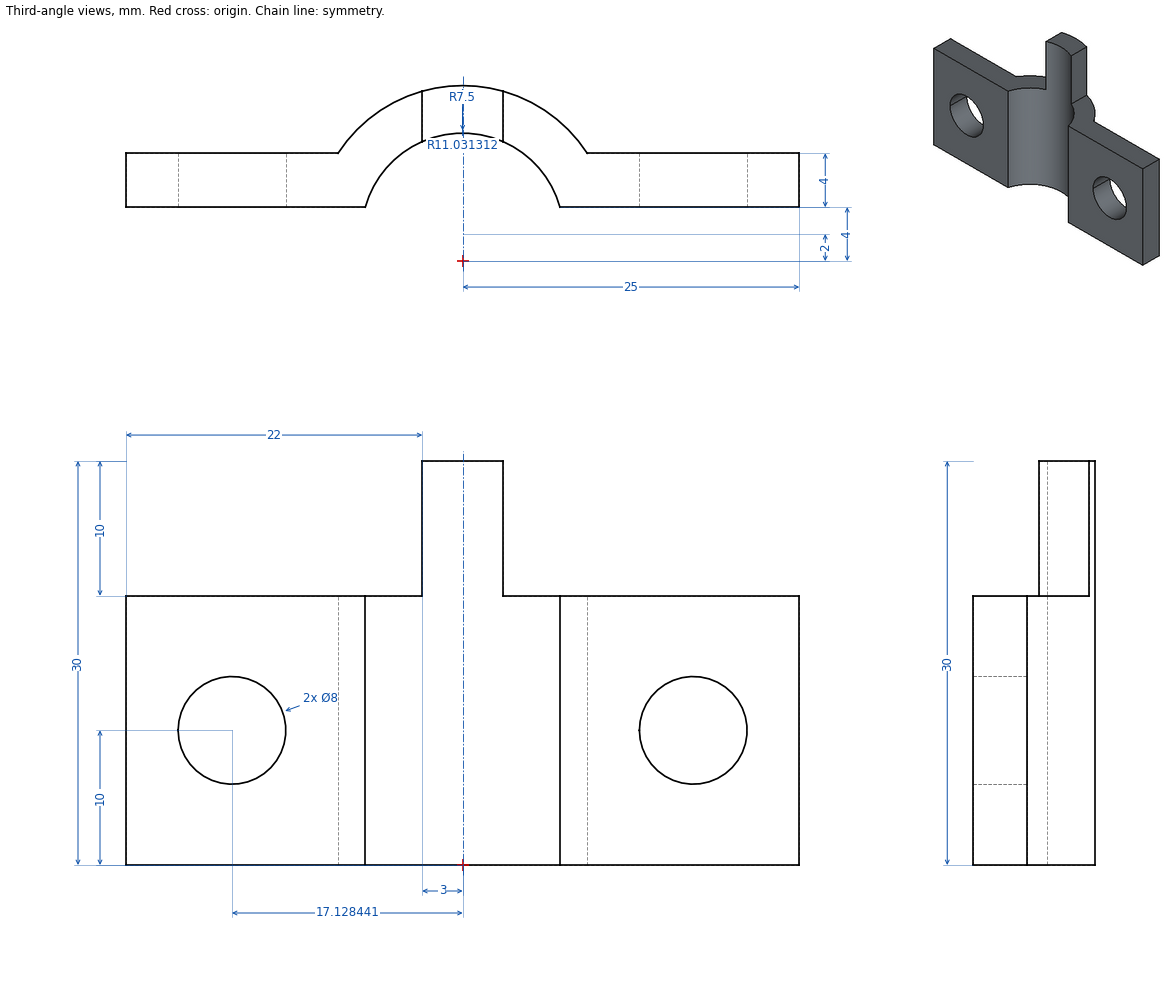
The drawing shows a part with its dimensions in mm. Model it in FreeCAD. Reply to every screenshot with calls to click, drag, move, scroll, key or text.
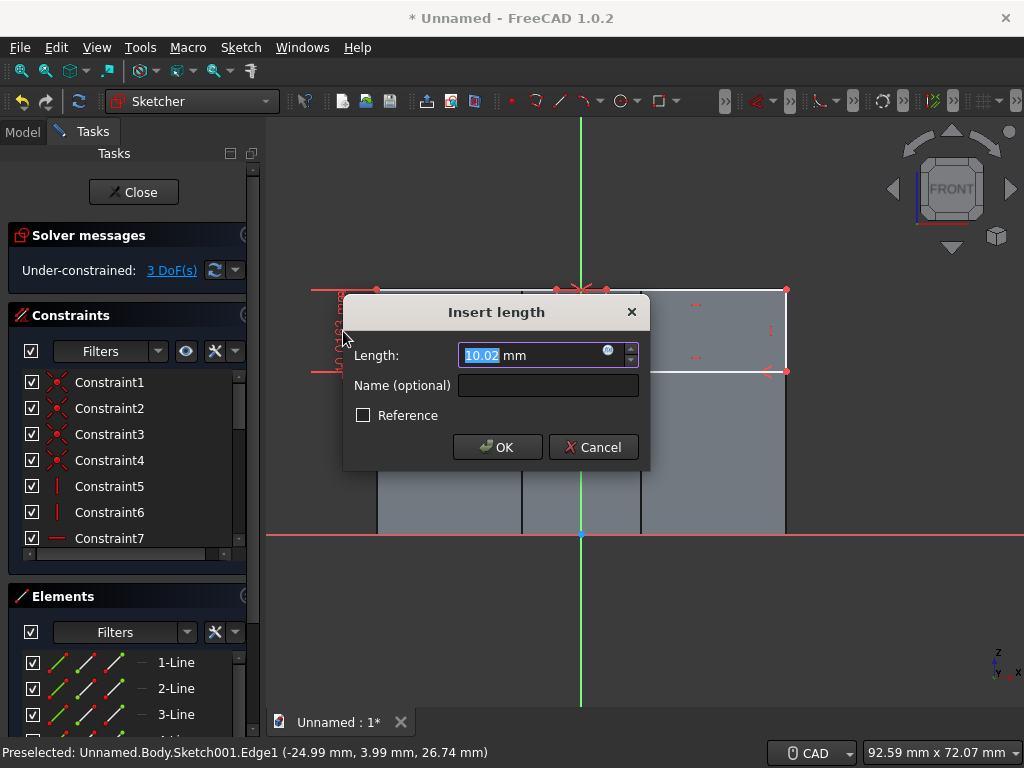
text(10)
key(Return)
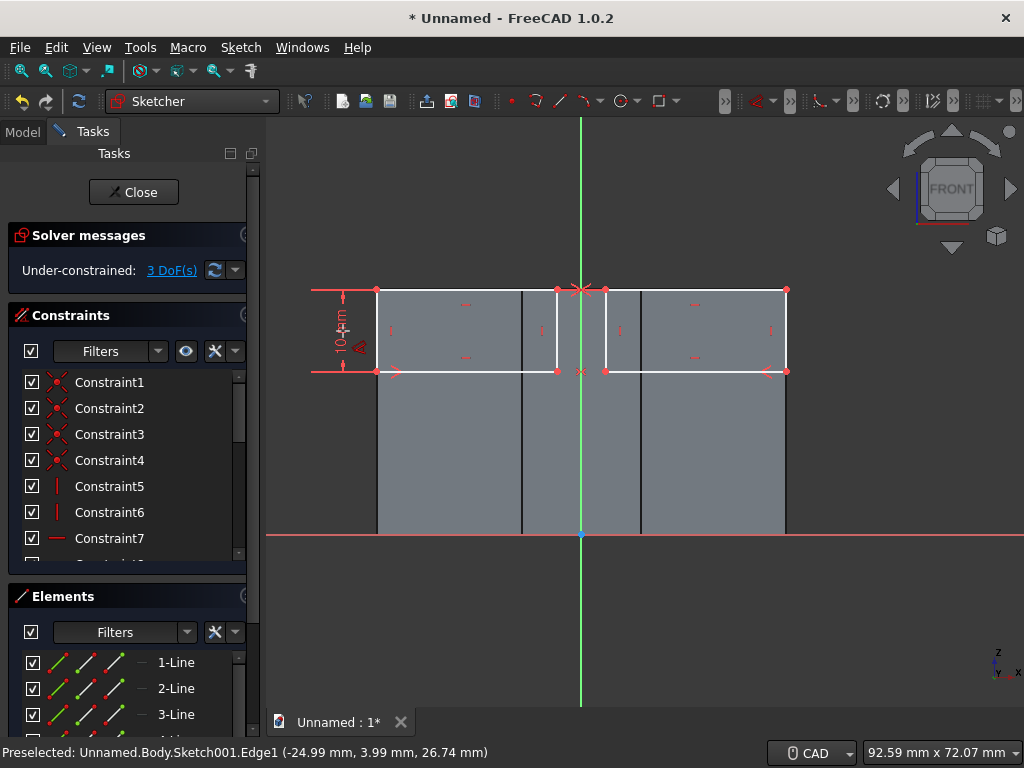
click(431, 372)
click(467, 338)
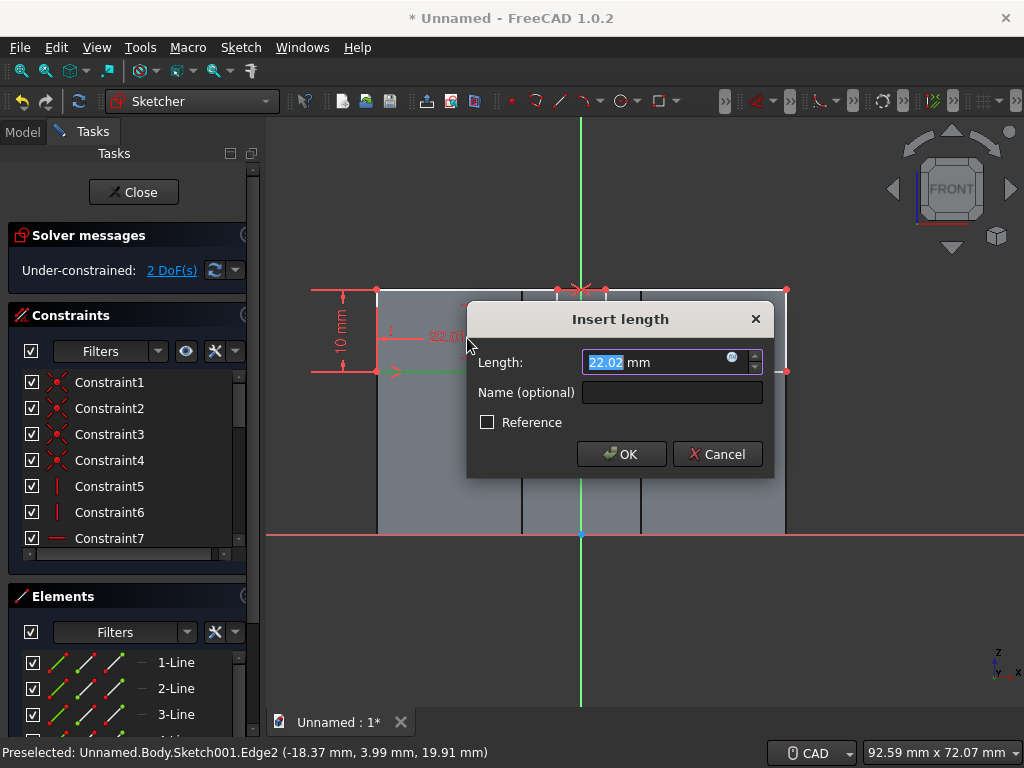
text(22)
key(Return)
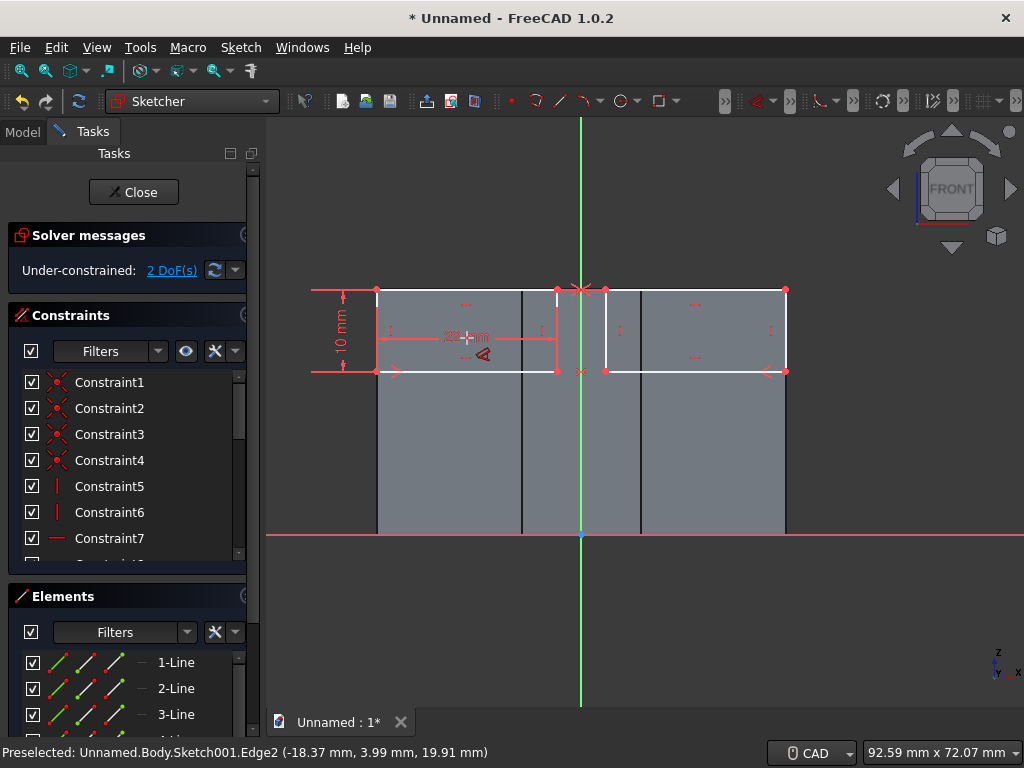
scroll(557, 372, up, 3)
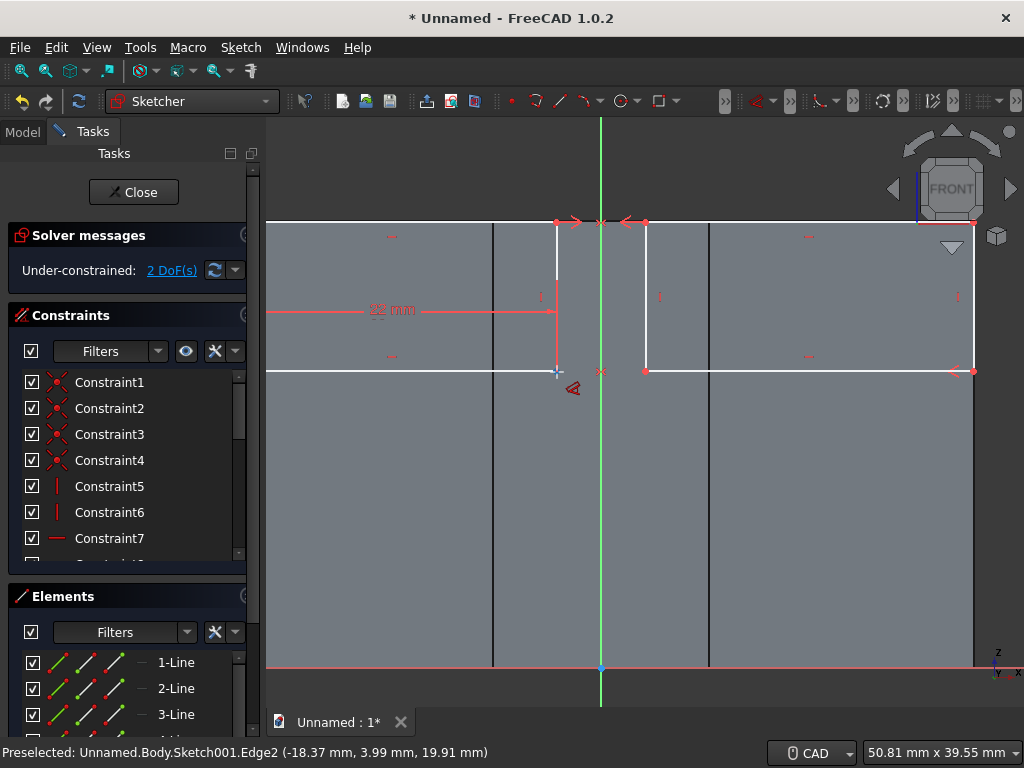
click(557, 371)
click(579, 337)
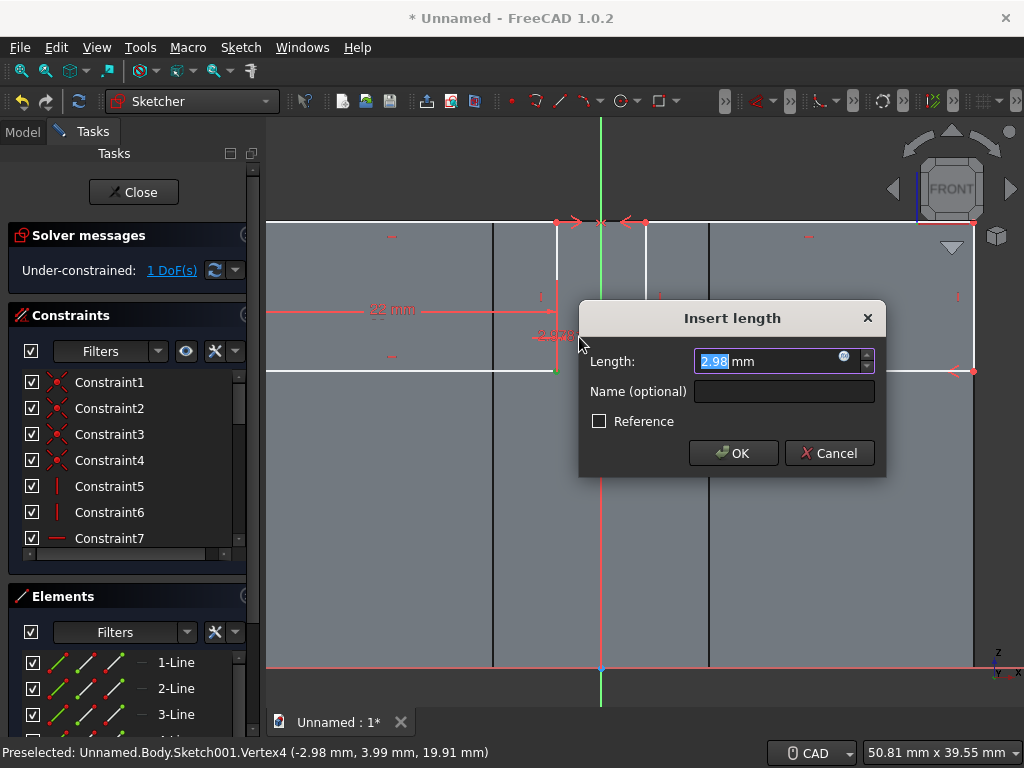
text(3)
key(Return)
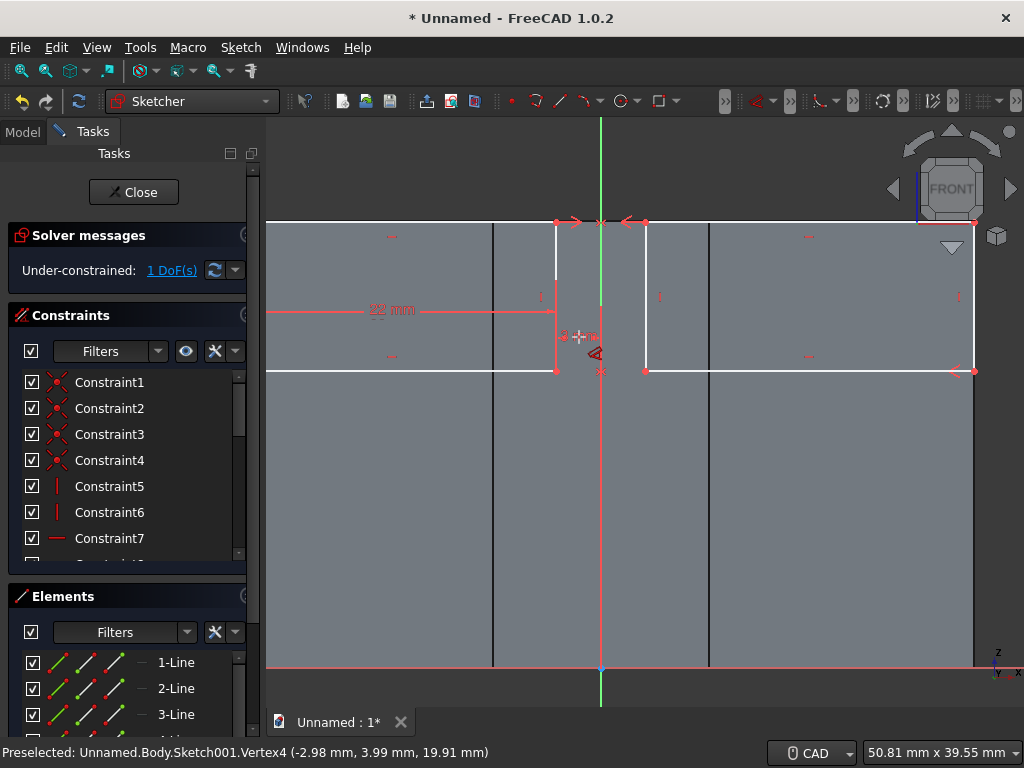
scroll(547, 372, down, 3)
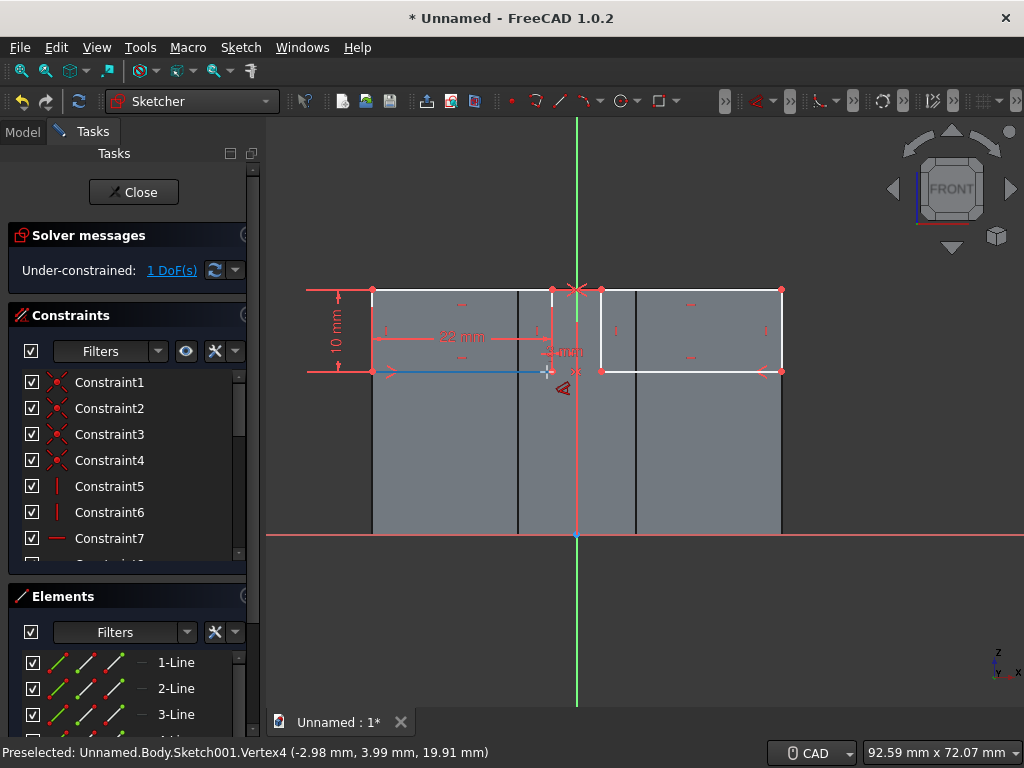
click(372, 290)
click(338, 412)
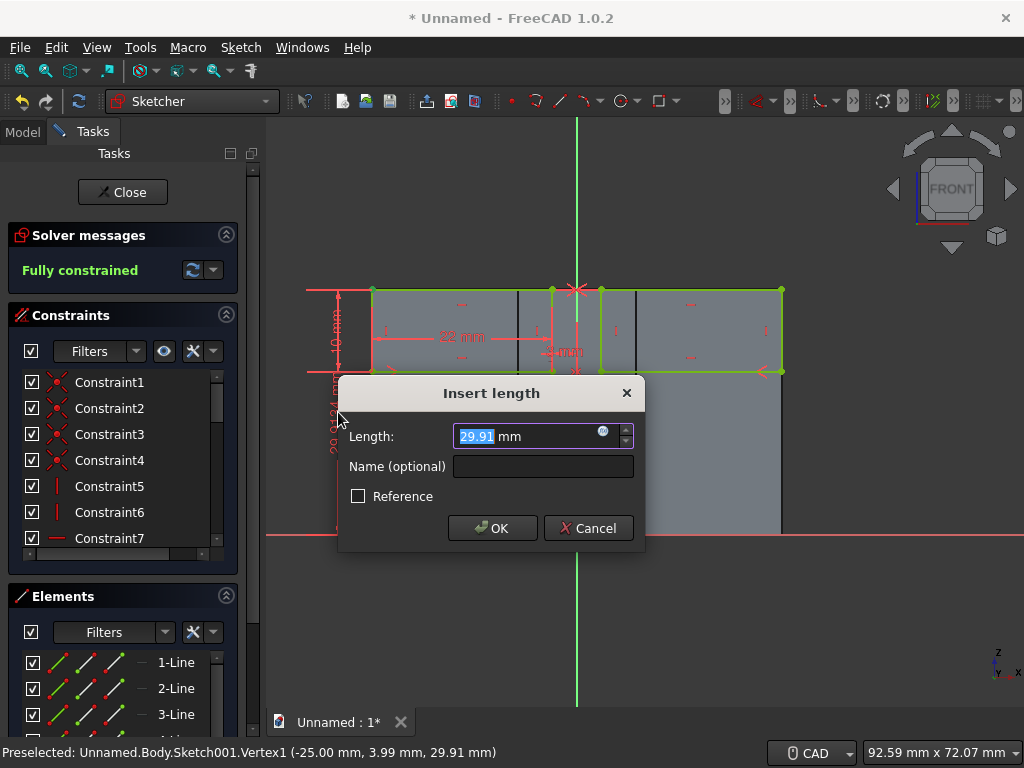
text(30)
key(Return)
key(Escape)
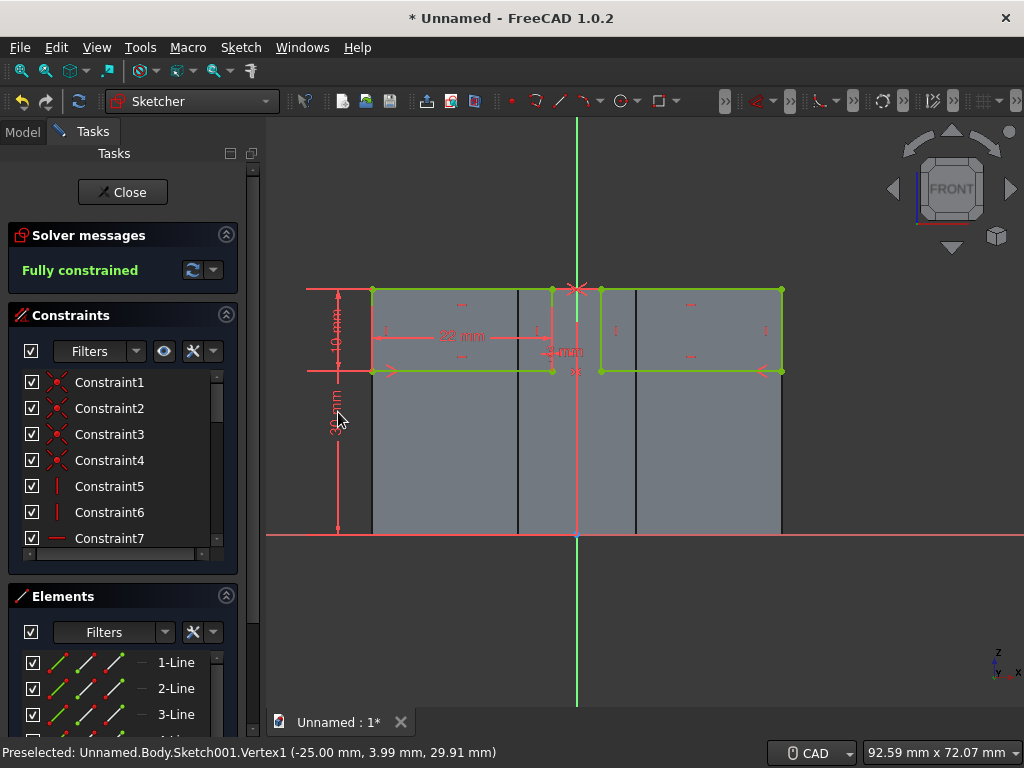
click(123, 192)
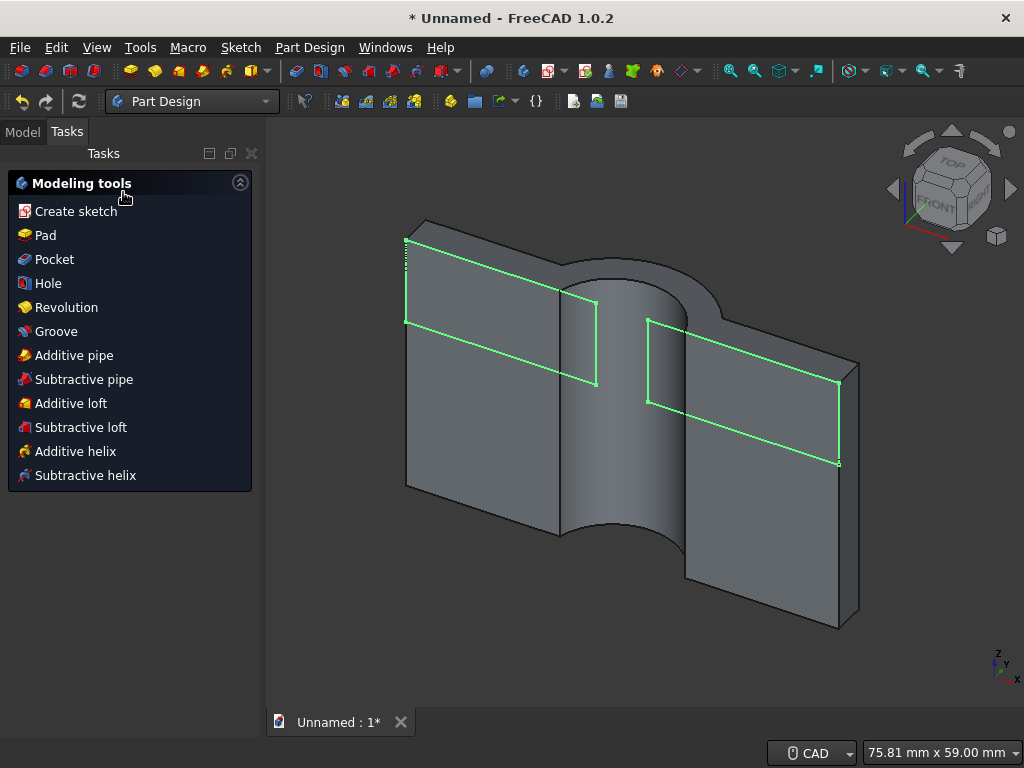
click(298, 72)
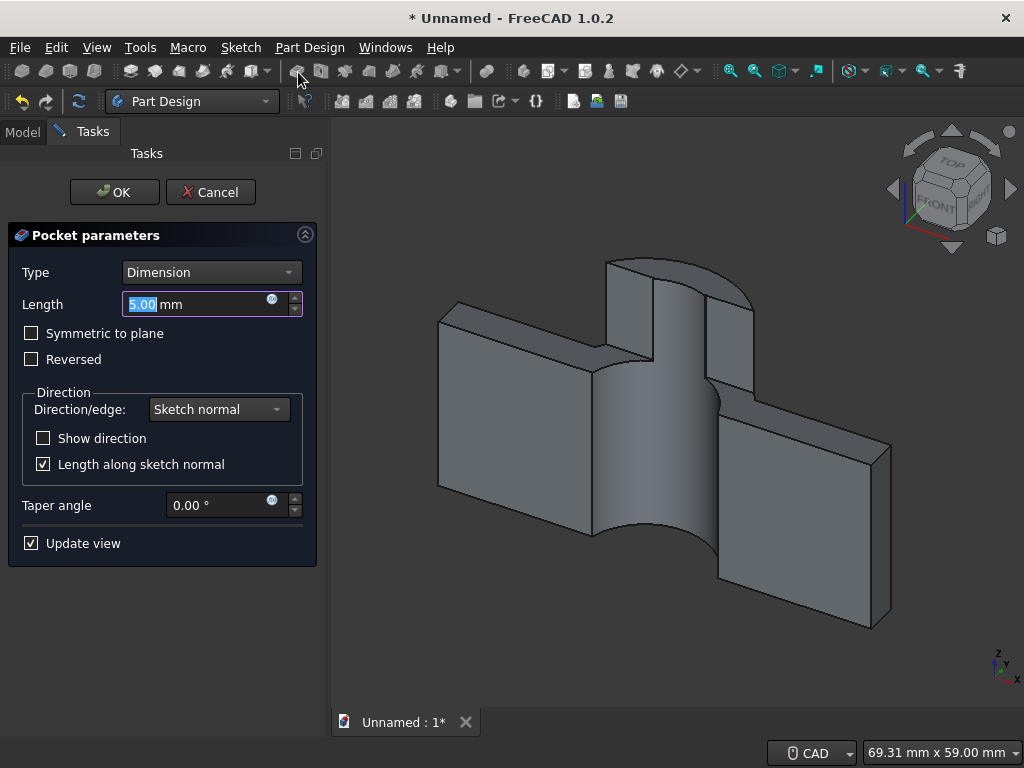
click(212, 272)